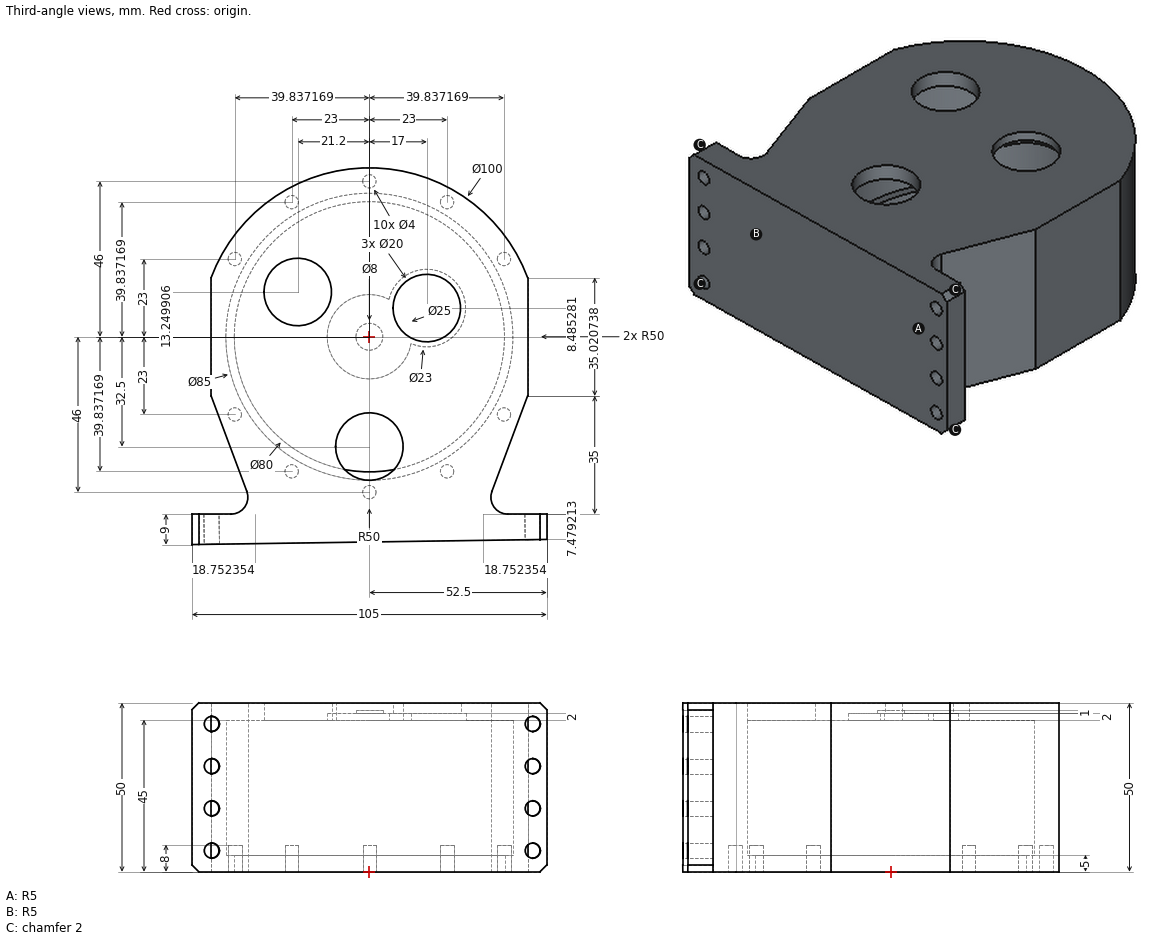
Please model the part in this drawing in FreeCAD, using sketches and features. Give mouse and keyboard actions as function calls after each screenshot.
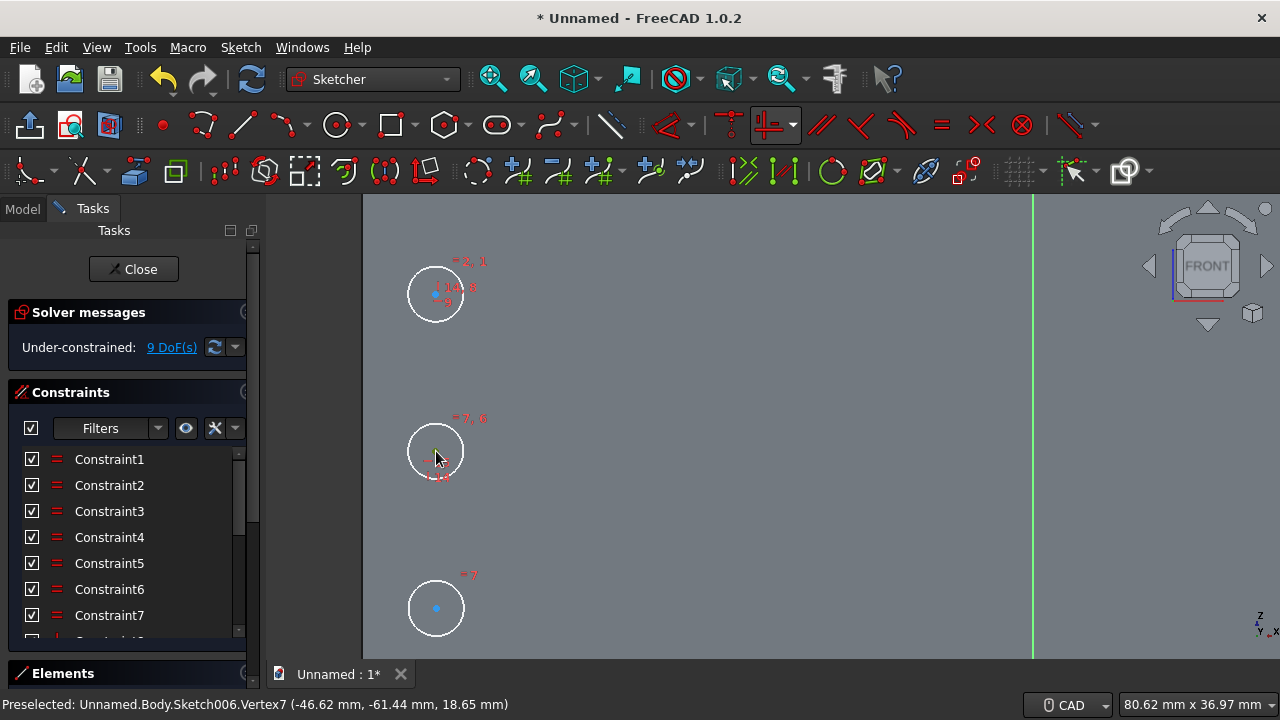
click(436, 608)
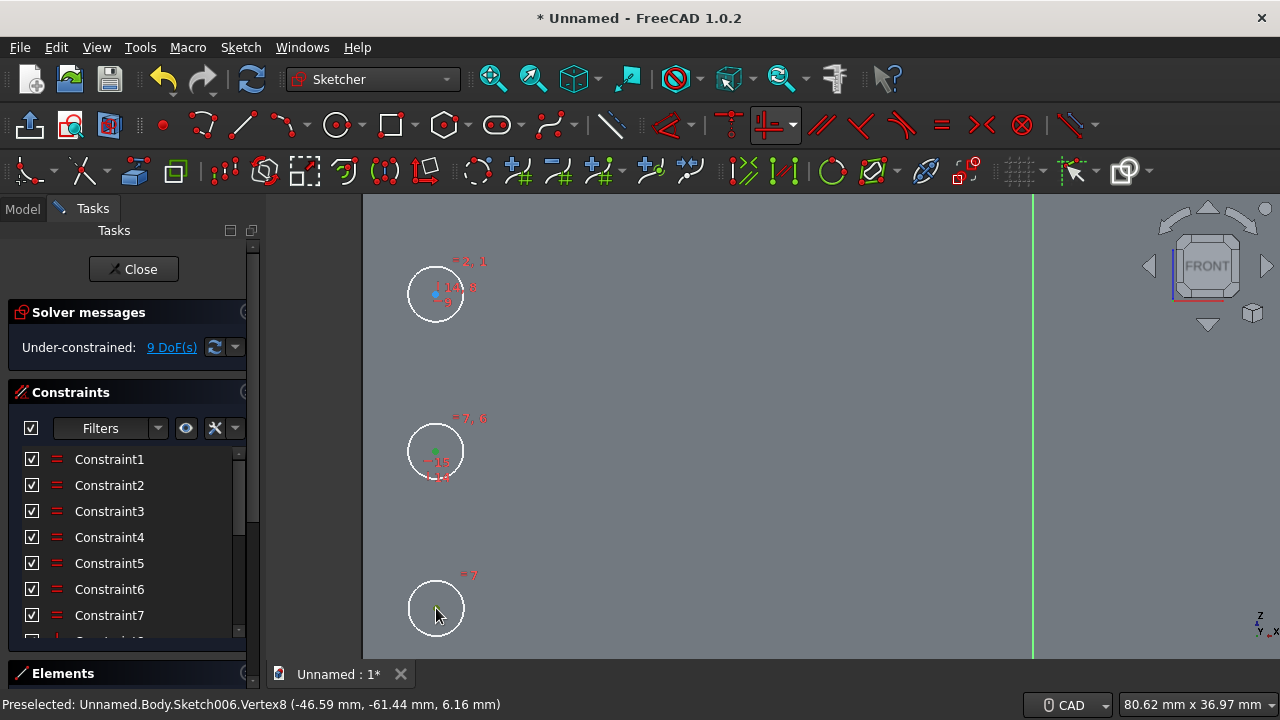
key(v)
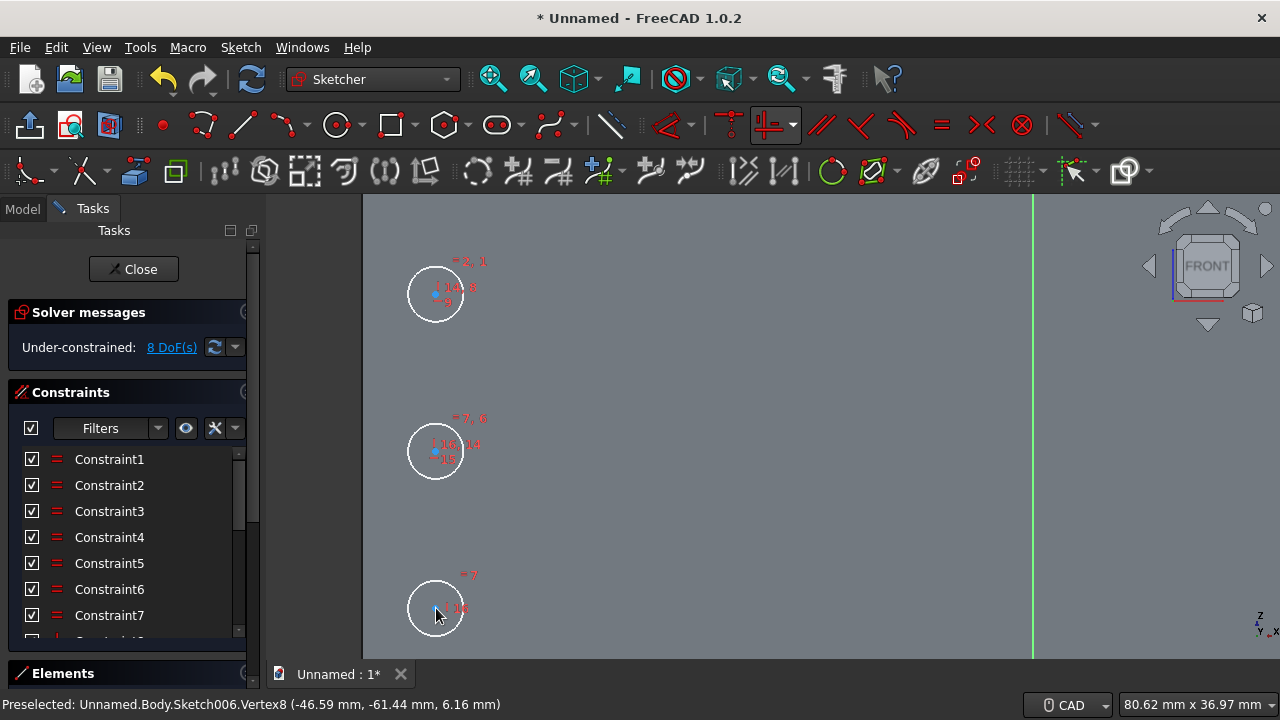
scroll(436, 451, down, 4)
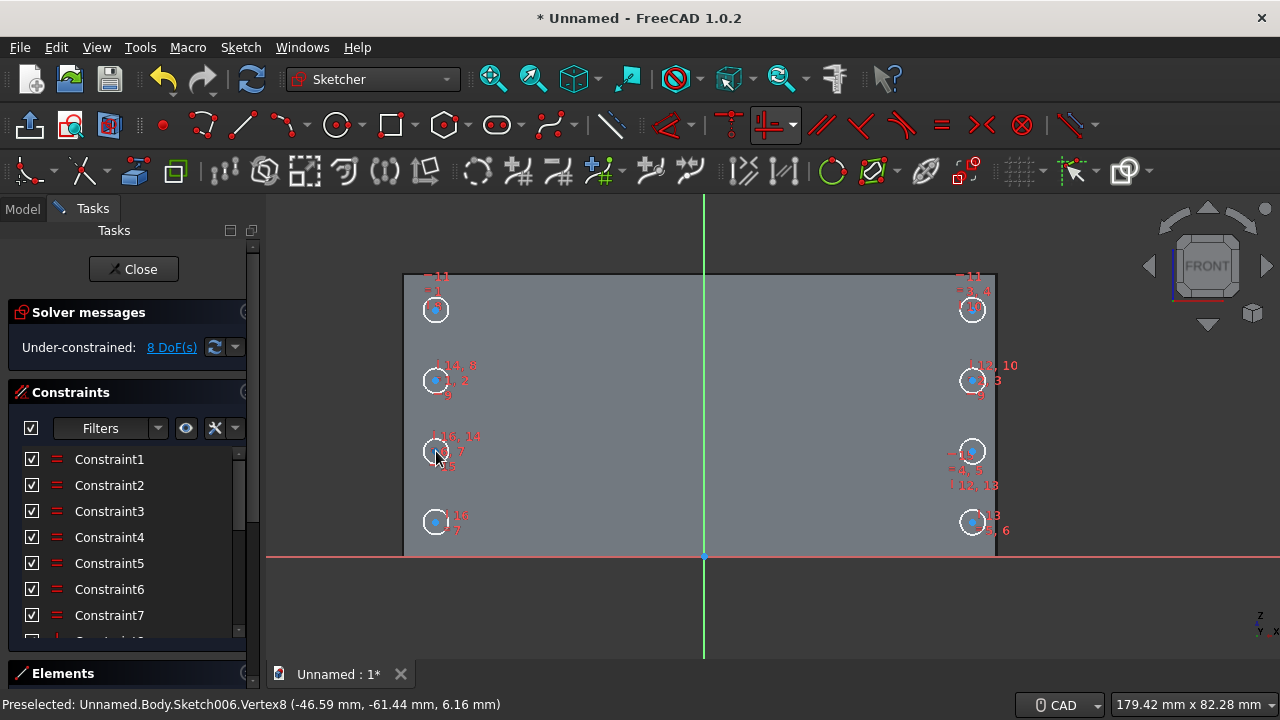
click(971, 524)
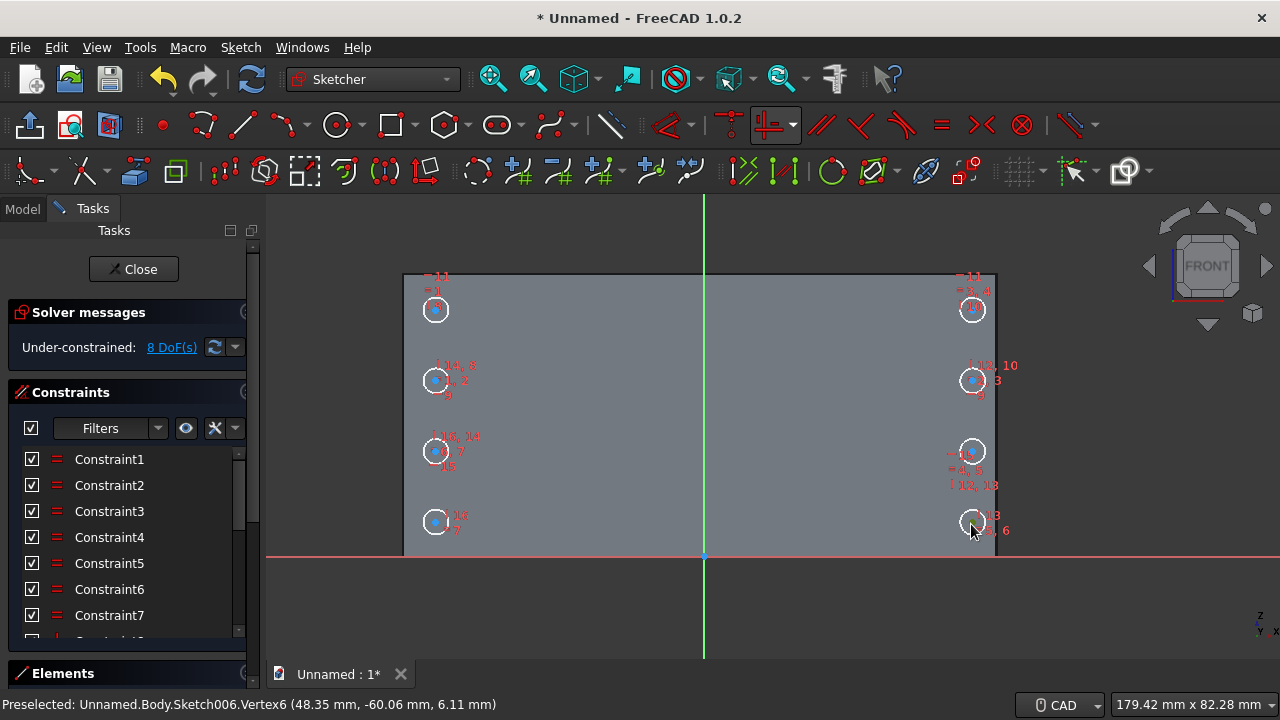
click(436, 522)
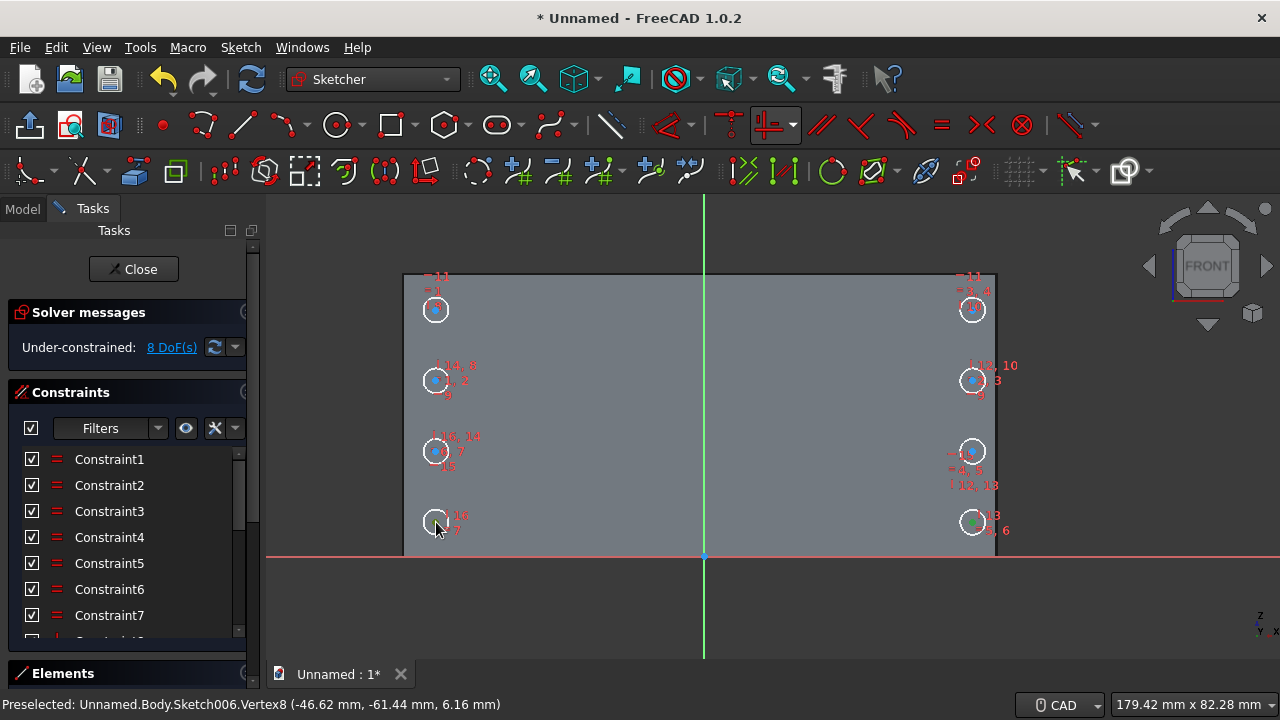
click(796, 126)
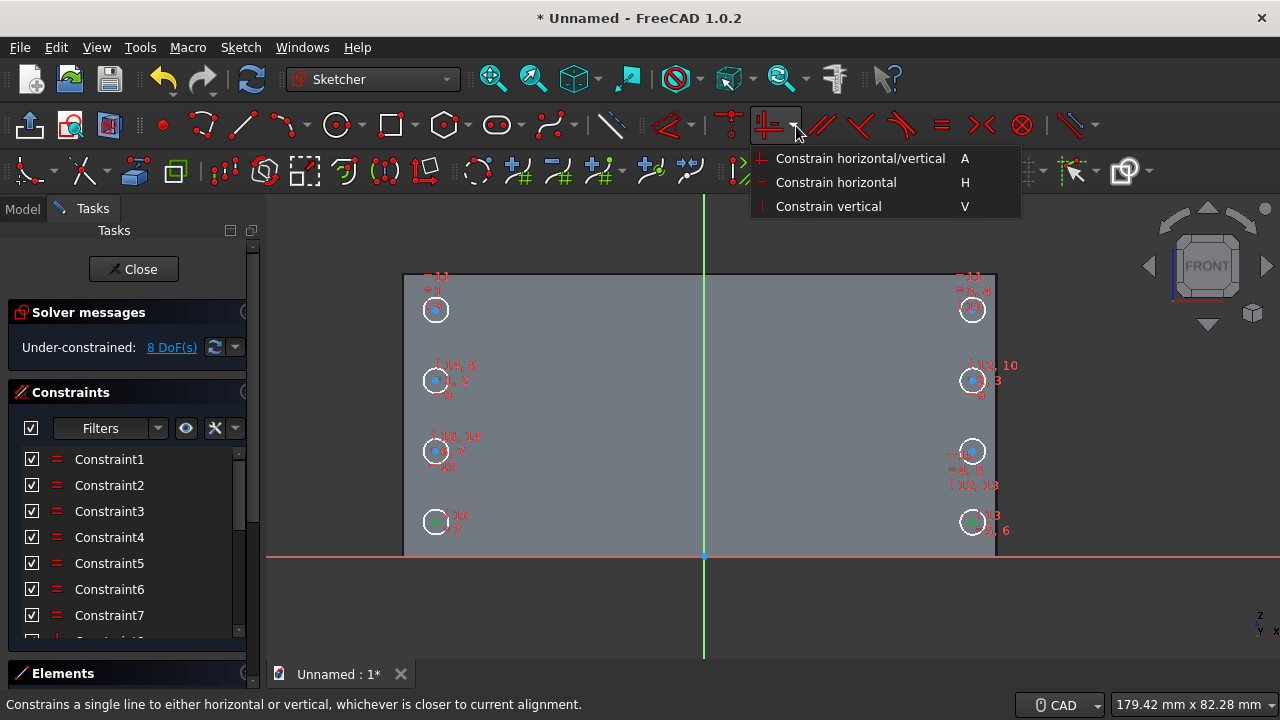
click(886, 182)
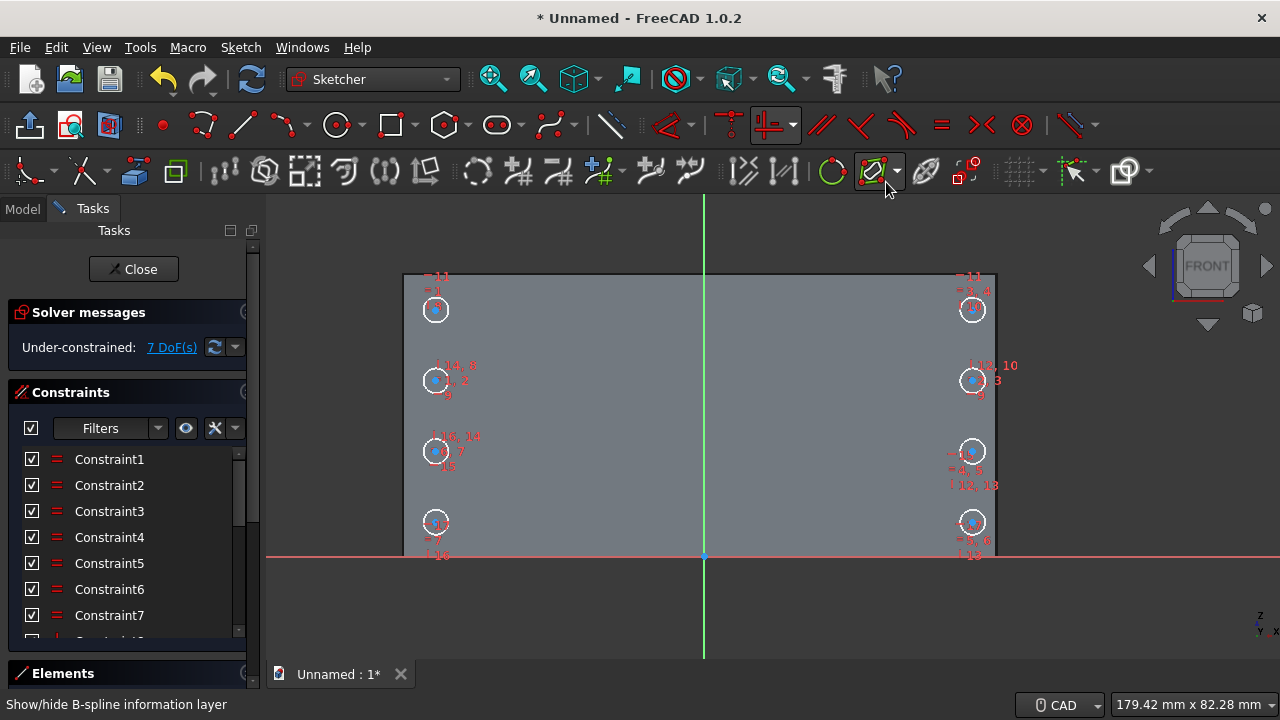
click(666, 126)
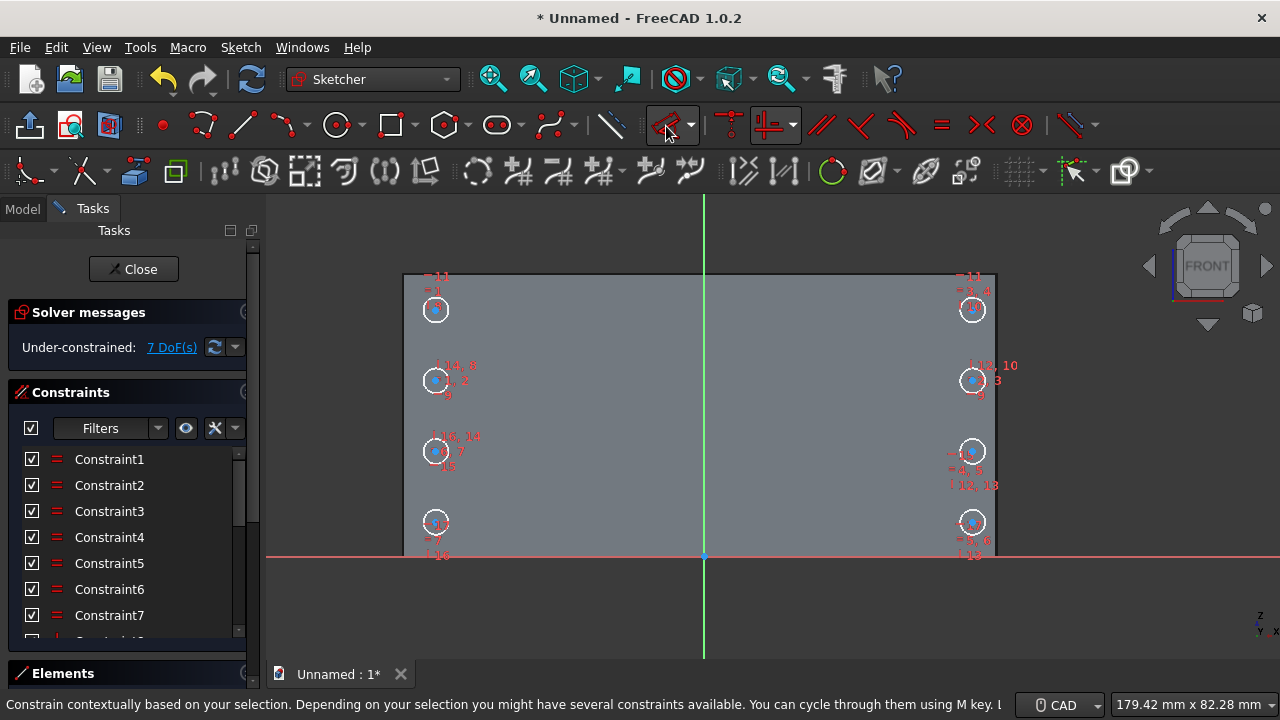
scroll(445, 301, up, 3)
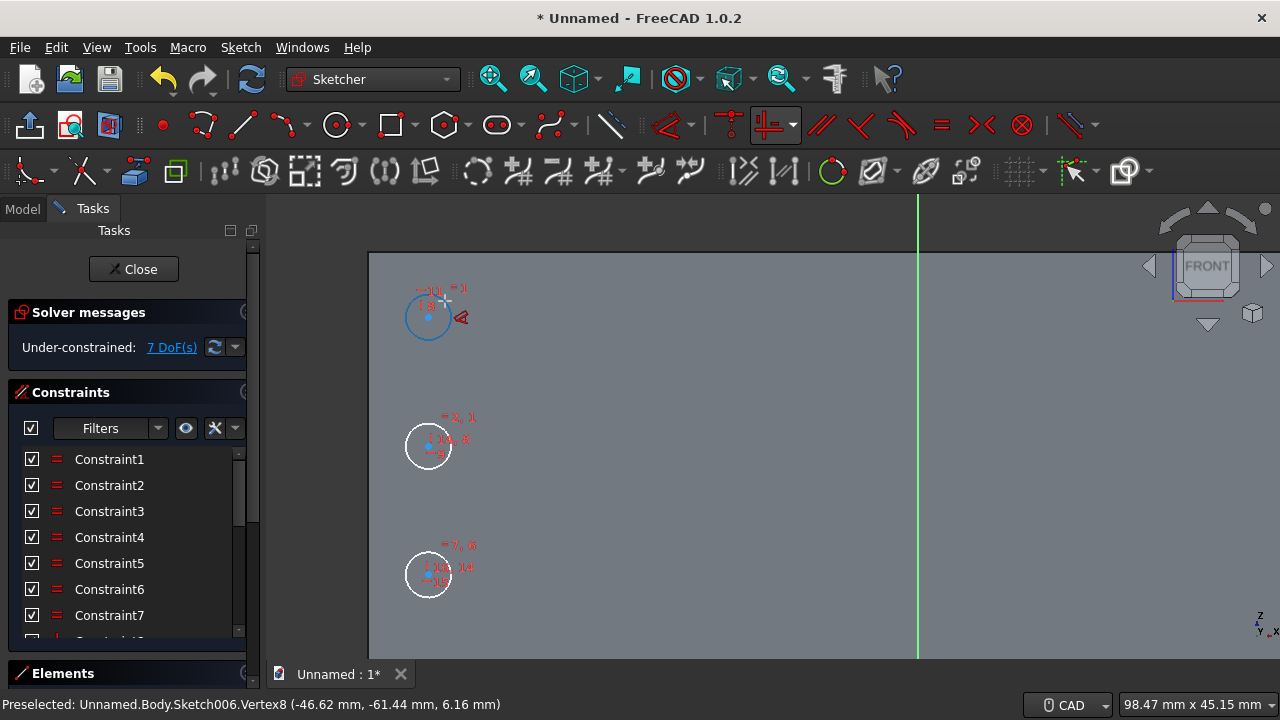
click(444, 301)
click(466, 278)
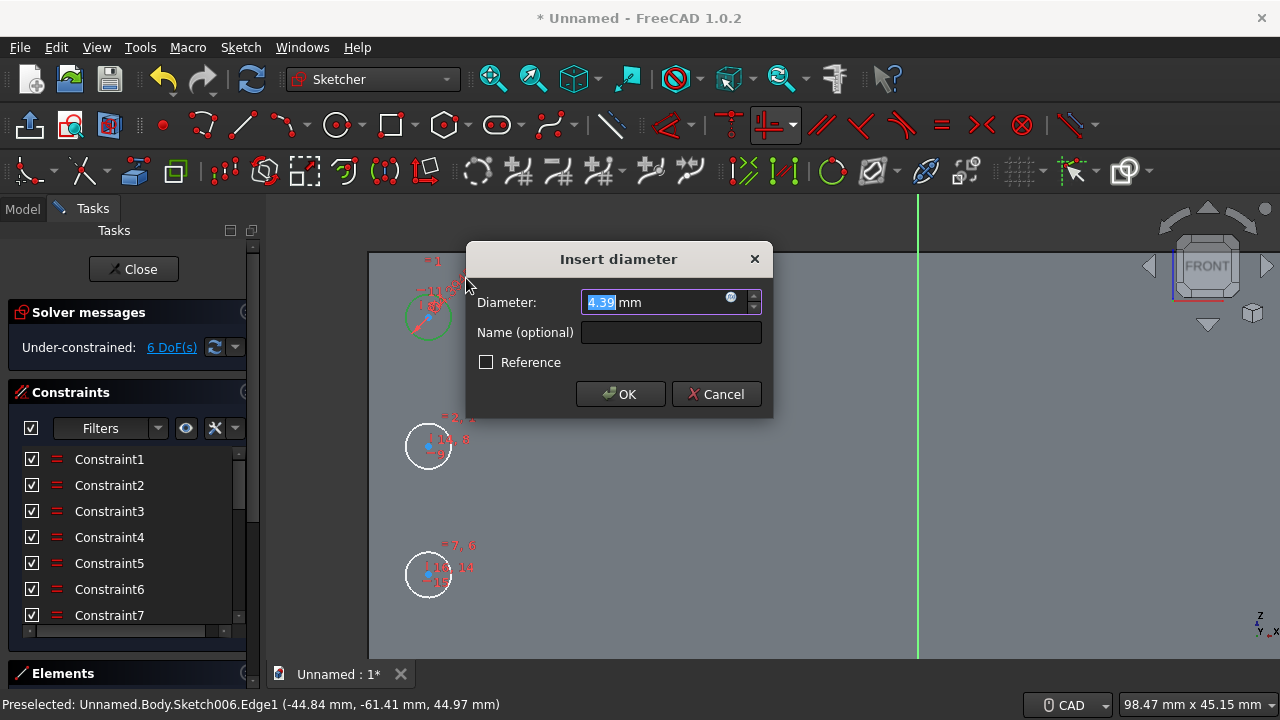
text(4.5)
key(Return)